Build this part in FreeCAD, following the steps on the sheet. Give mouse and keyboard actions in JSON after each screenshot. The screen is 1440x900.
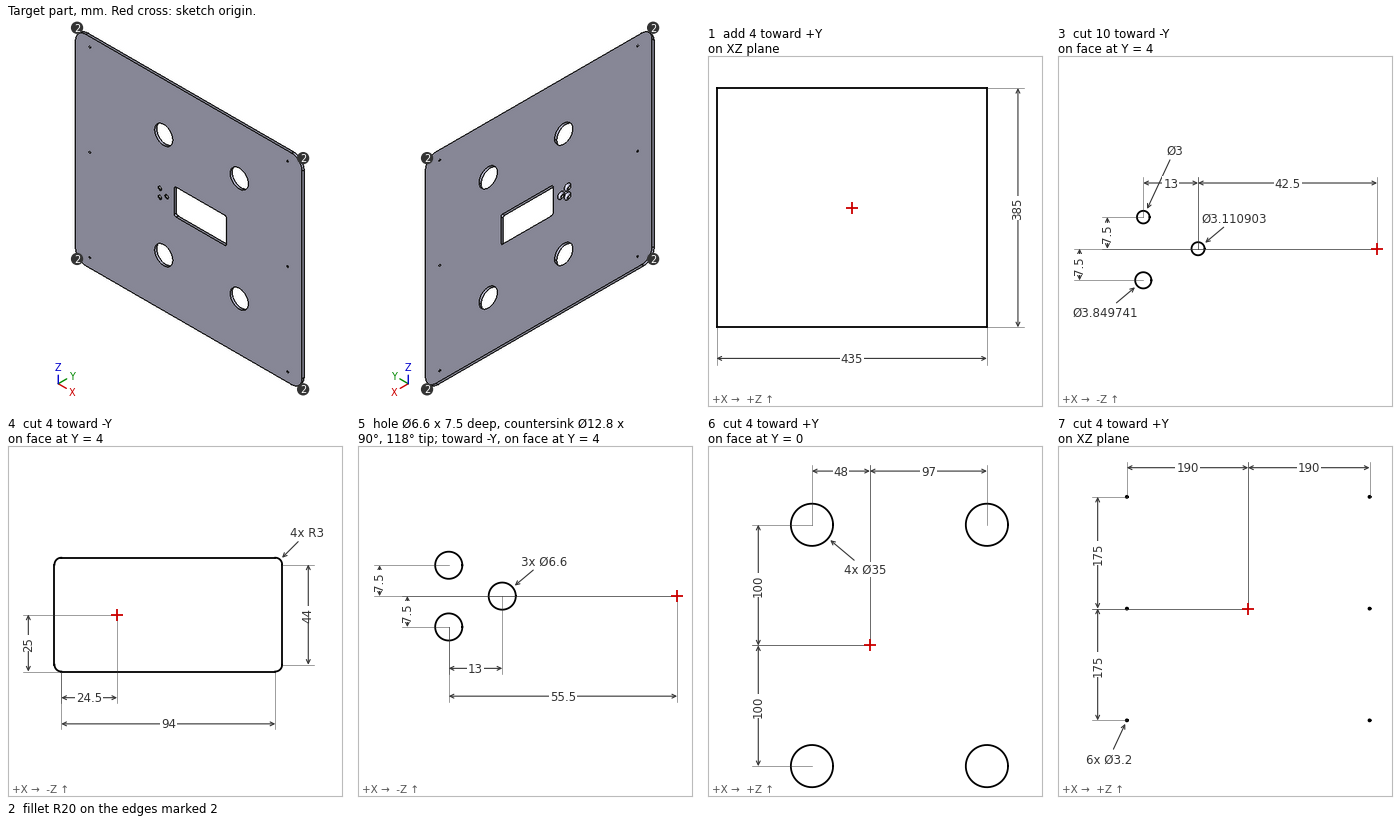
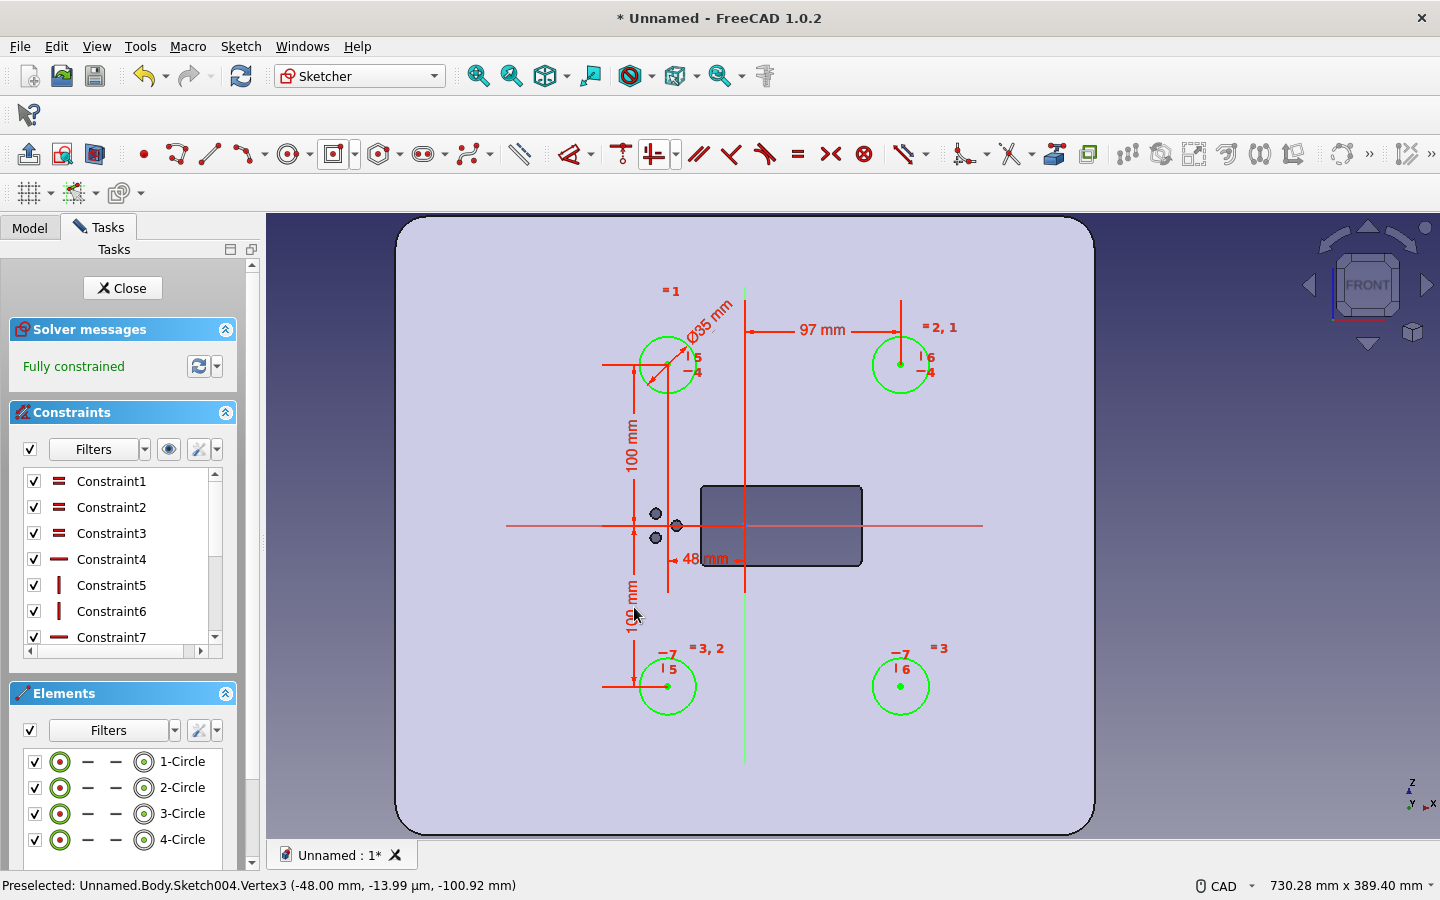
{"action": "left_click", "coordinate": [123, 288]}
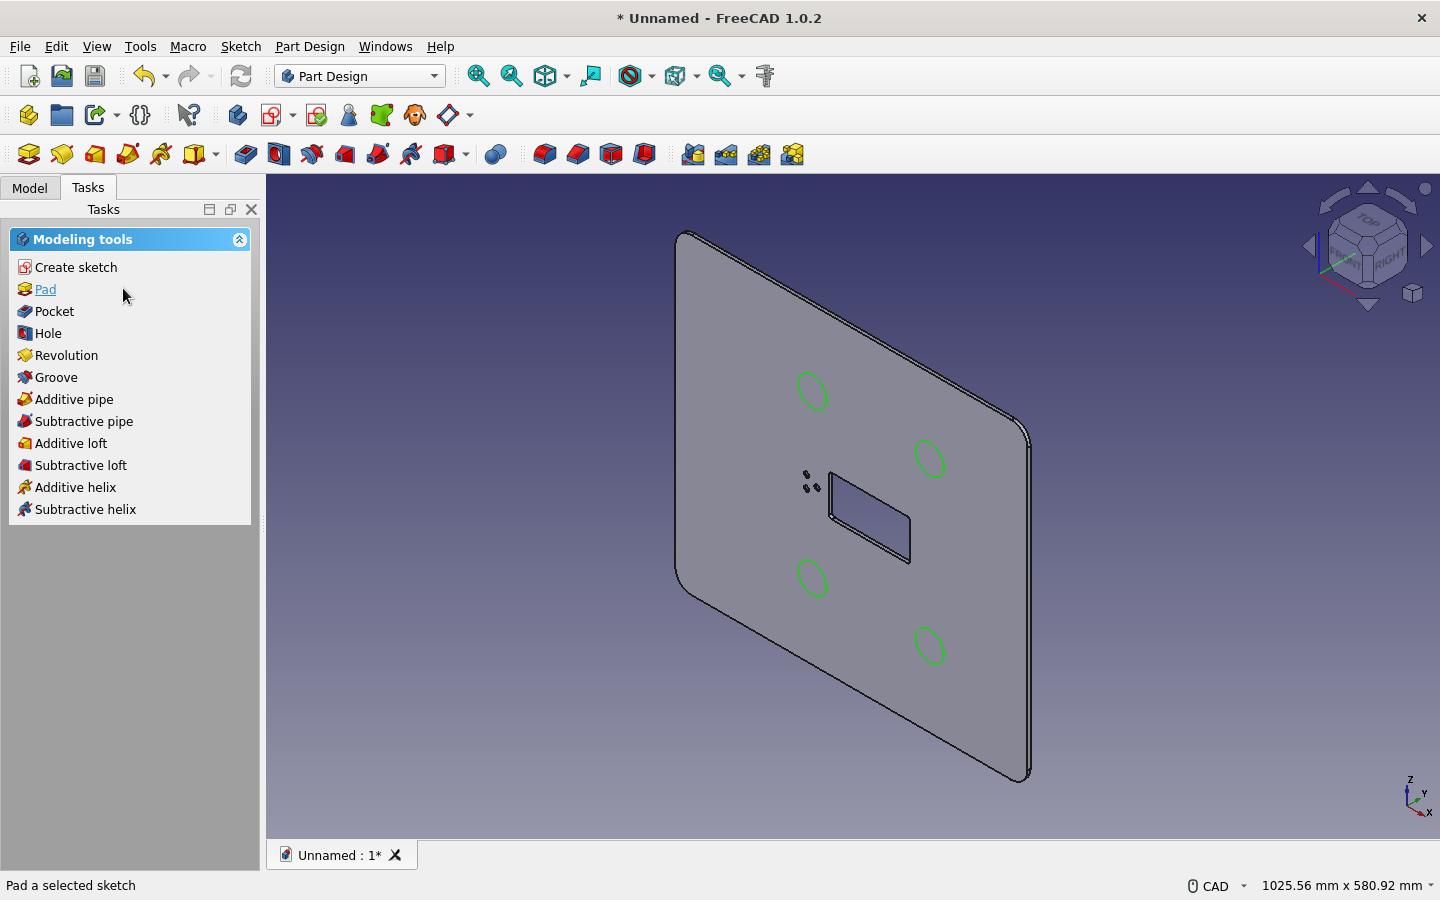
{"action": "left_click", "coordinate": [246, 154]}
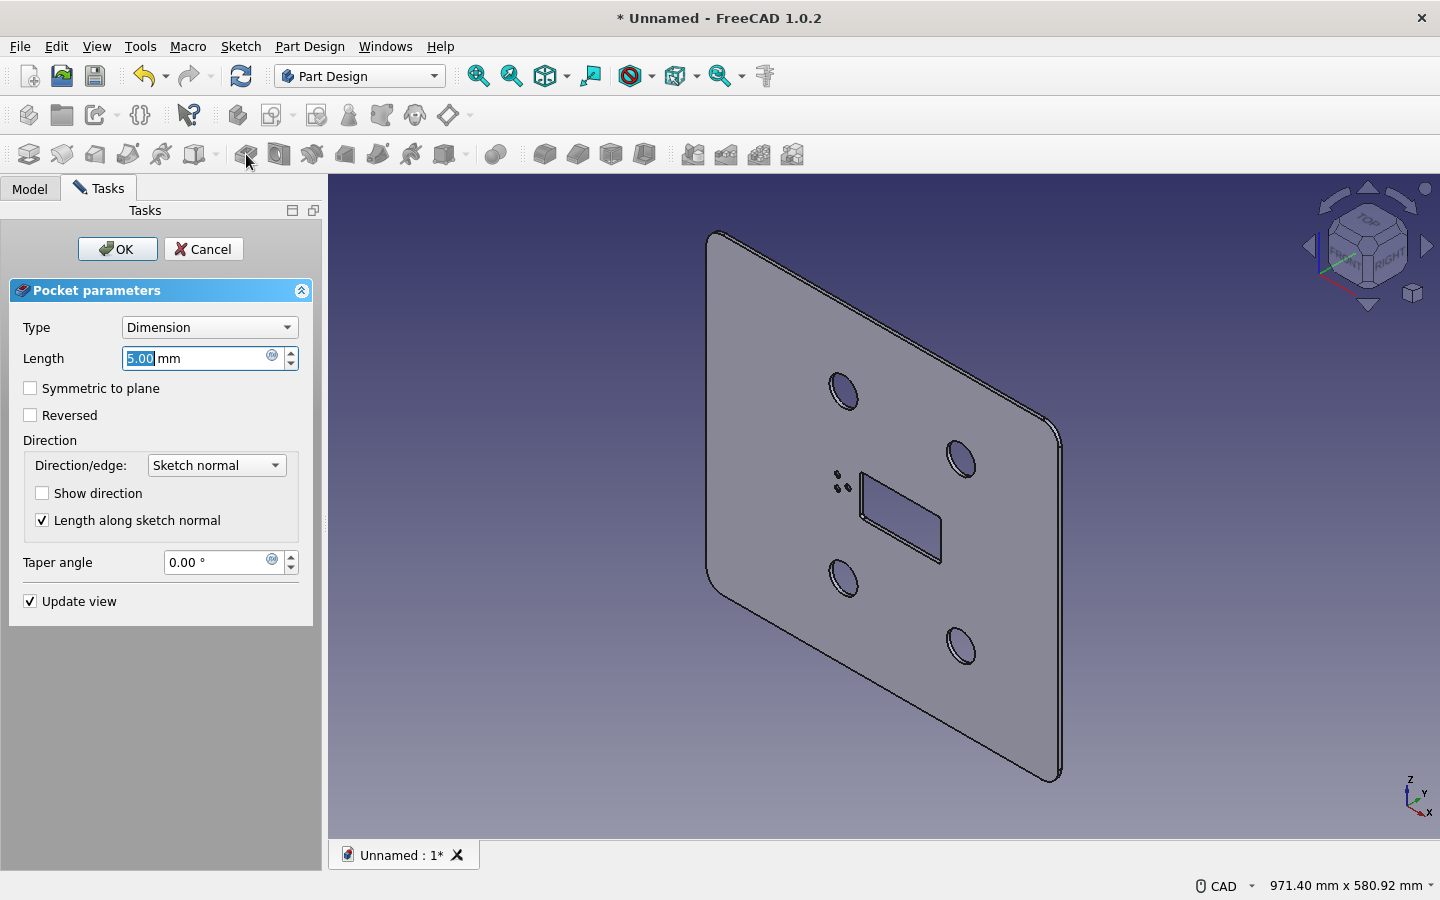
{"action": "type", "text": "4"}
{"action": "key", "text": "Tab"}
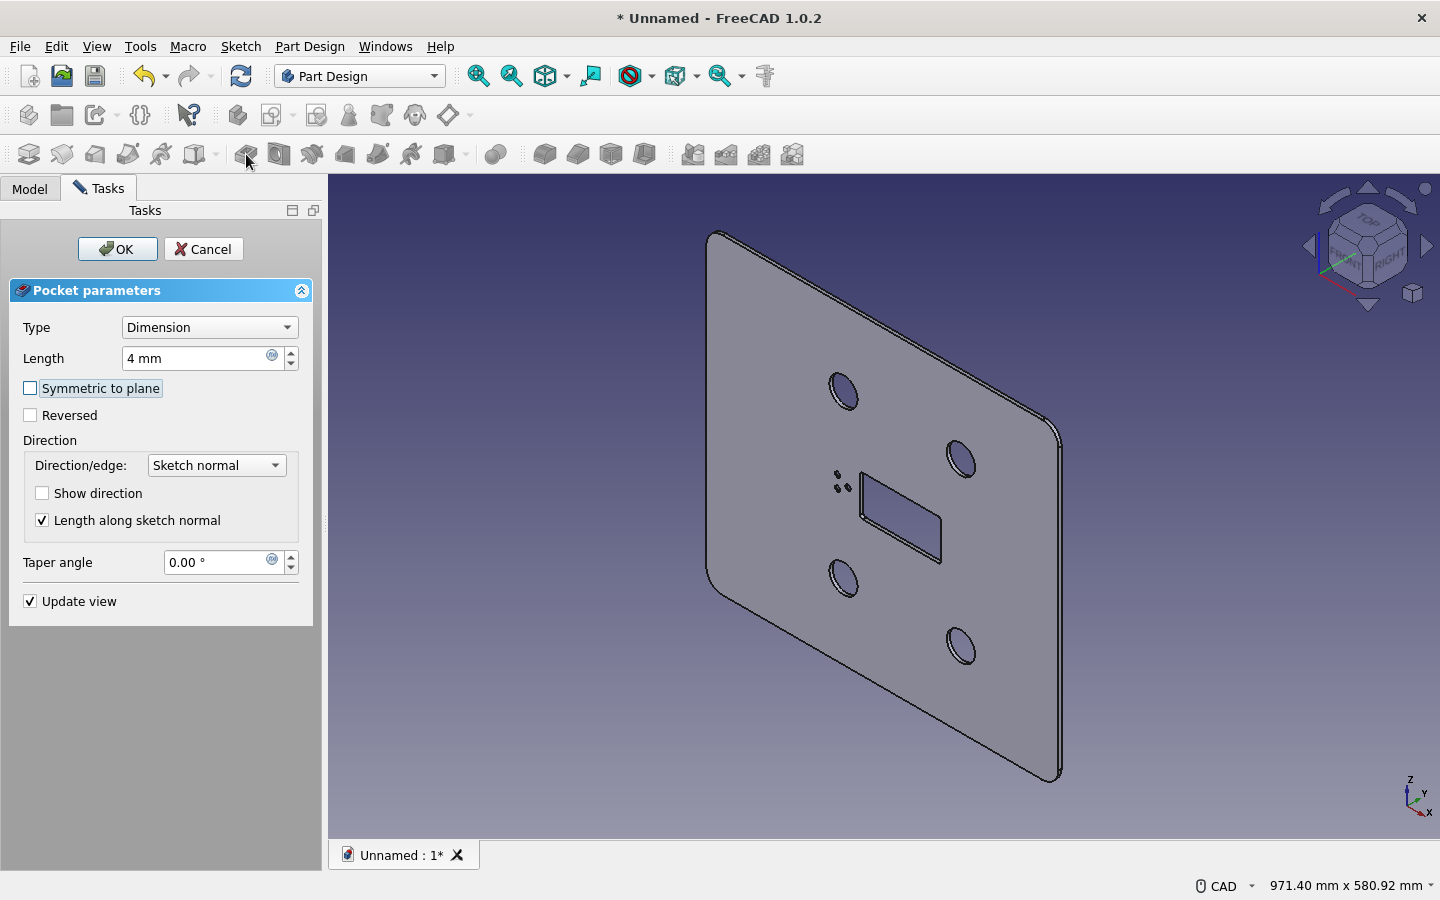
{"action": "left_click", "coordinate": [118, 249]}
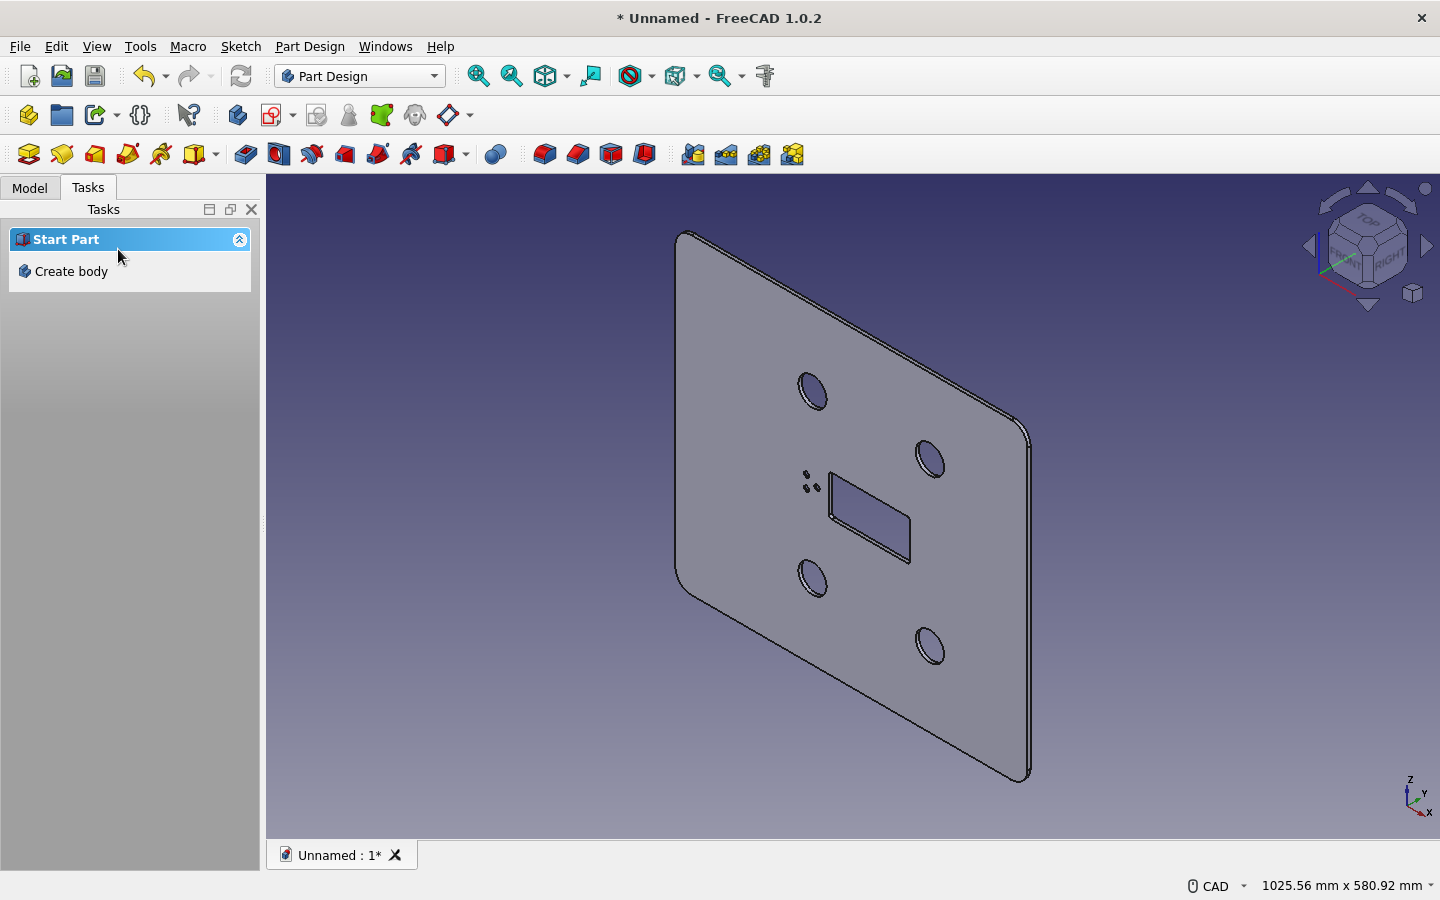
{"action": "left_click", "coordinate": [270, 116]}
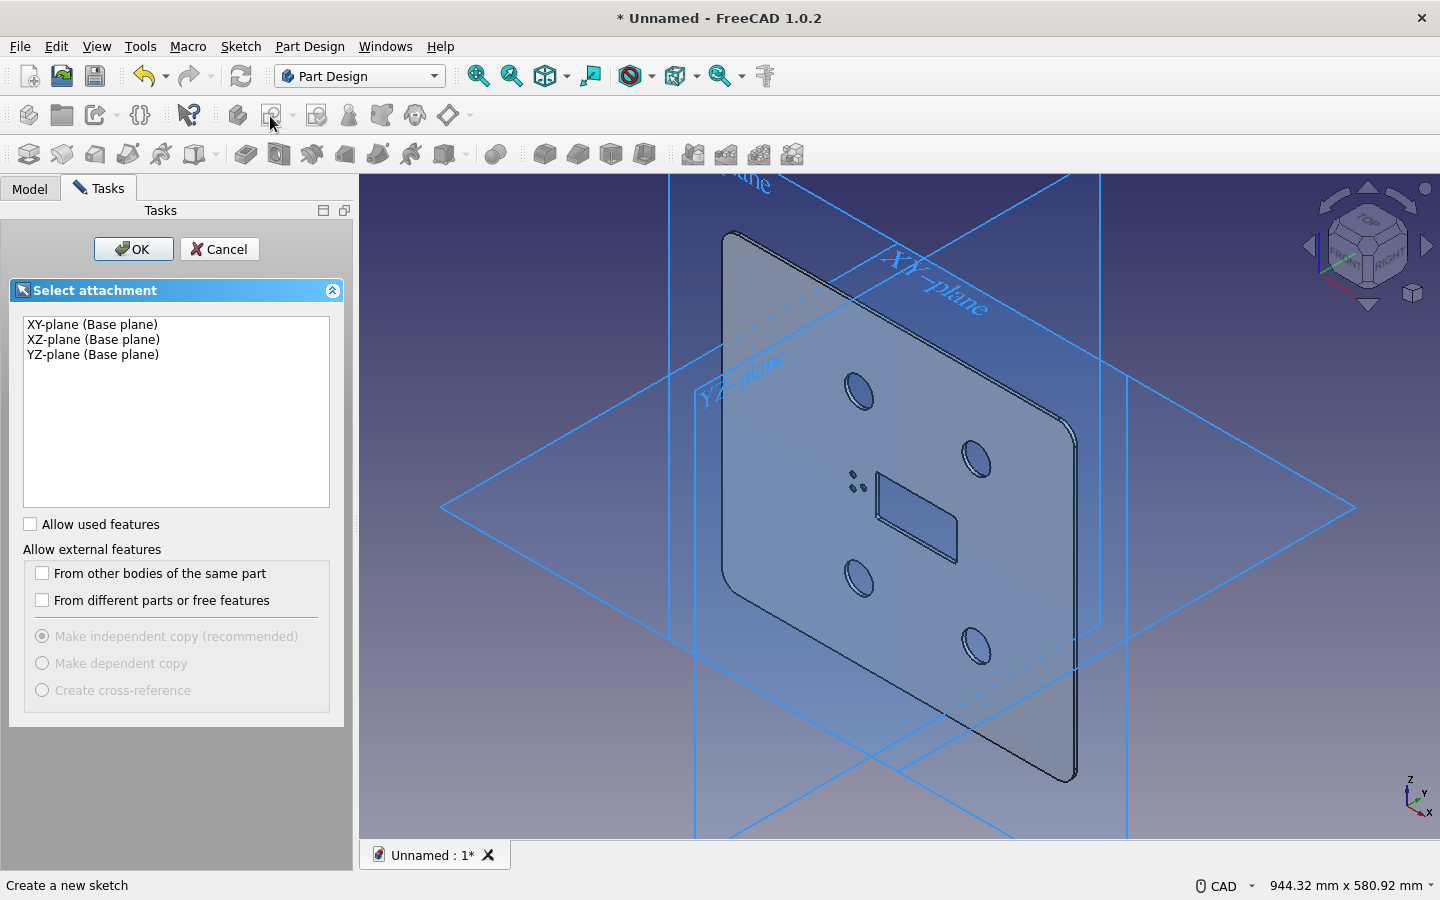
{"action": "left_click", "coordinate": [84, 340]}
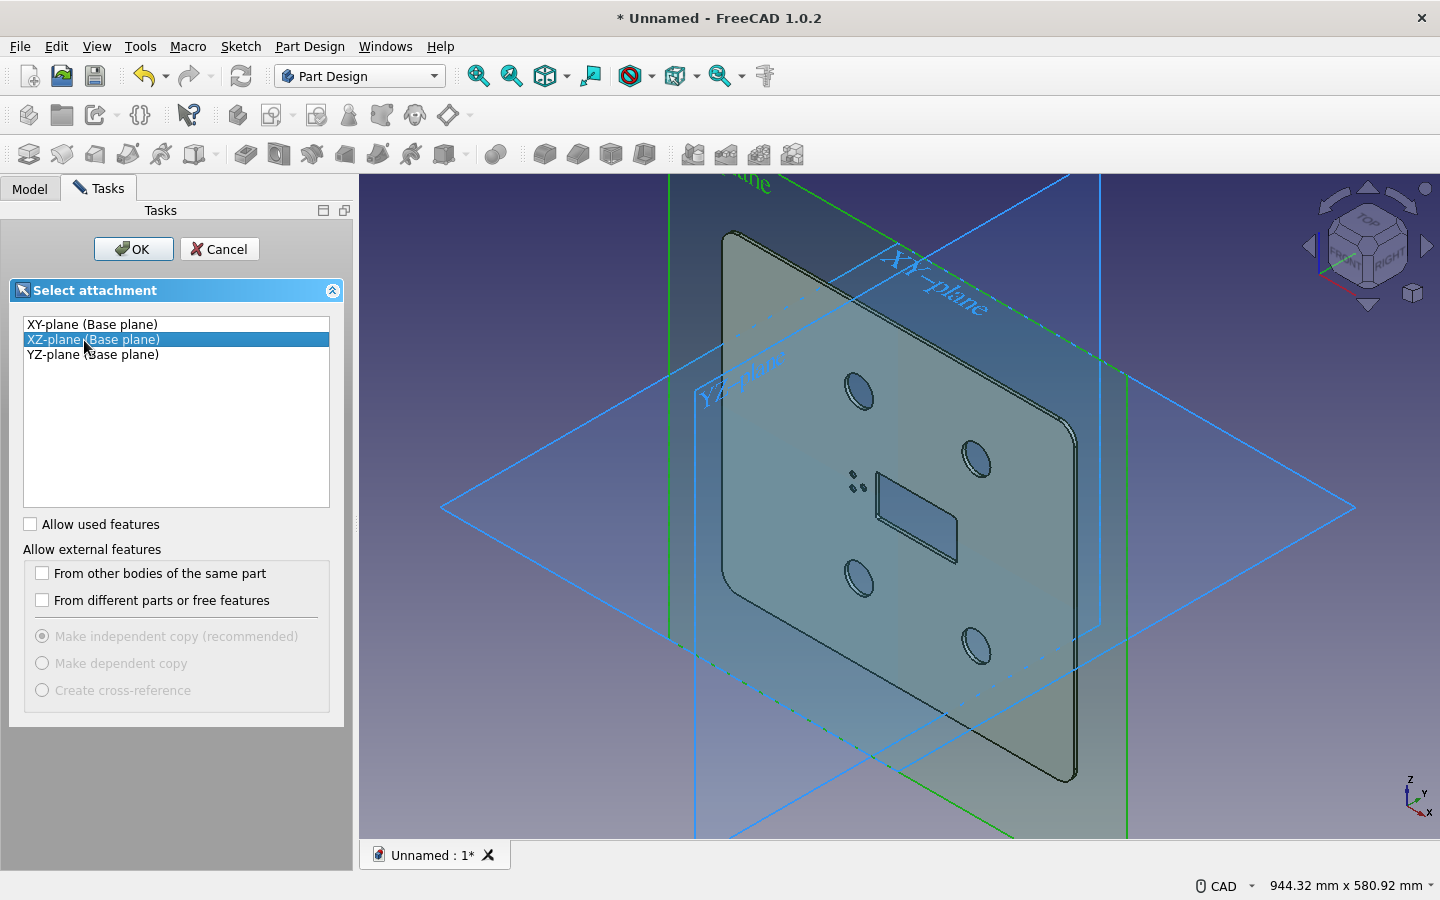
{"action": "left_click", "coordinate": [134, 249]}